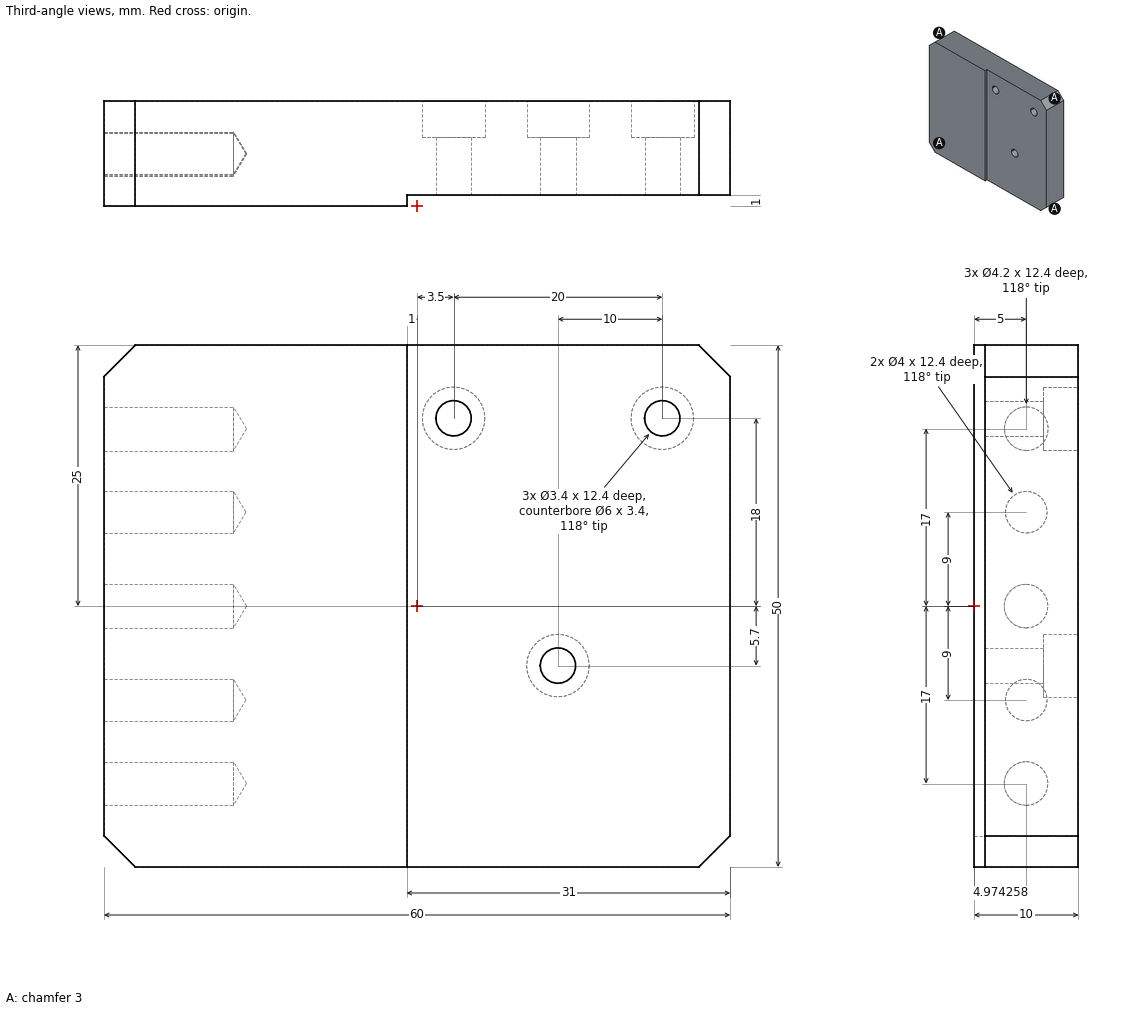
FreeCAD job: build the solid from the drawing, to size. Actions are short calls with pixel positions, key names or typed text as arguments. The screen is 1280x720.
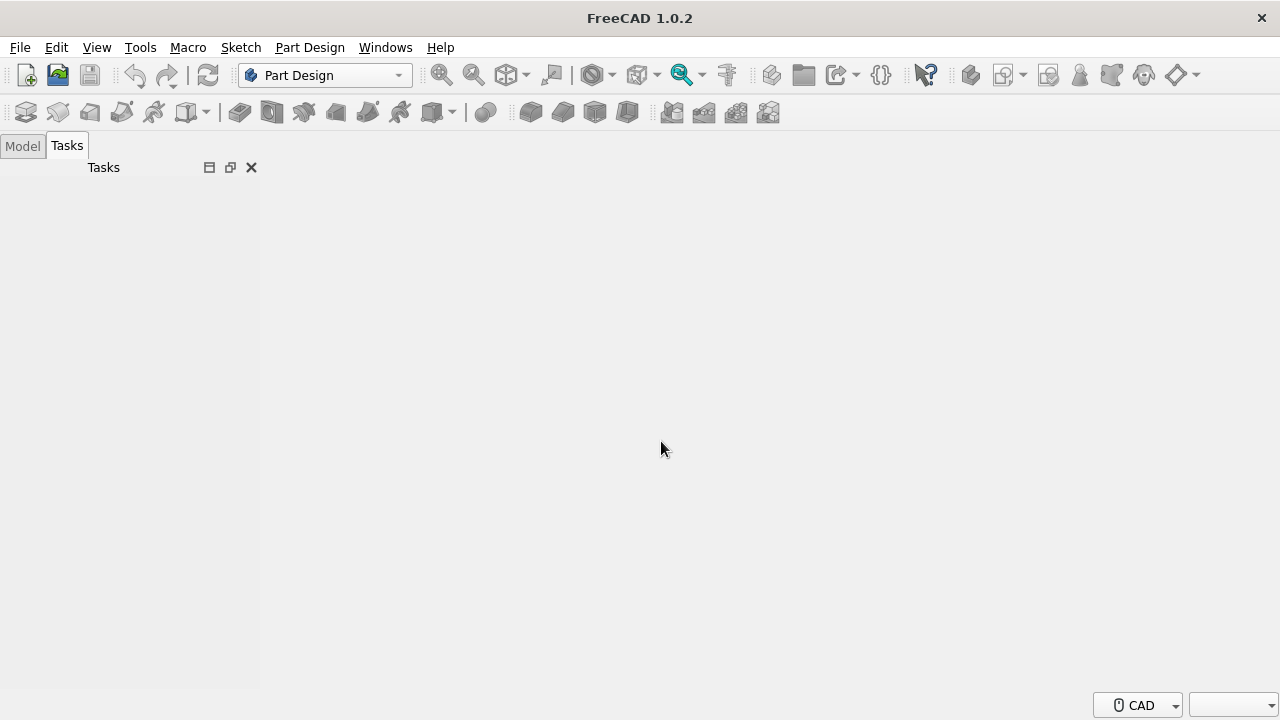
click(26, 76)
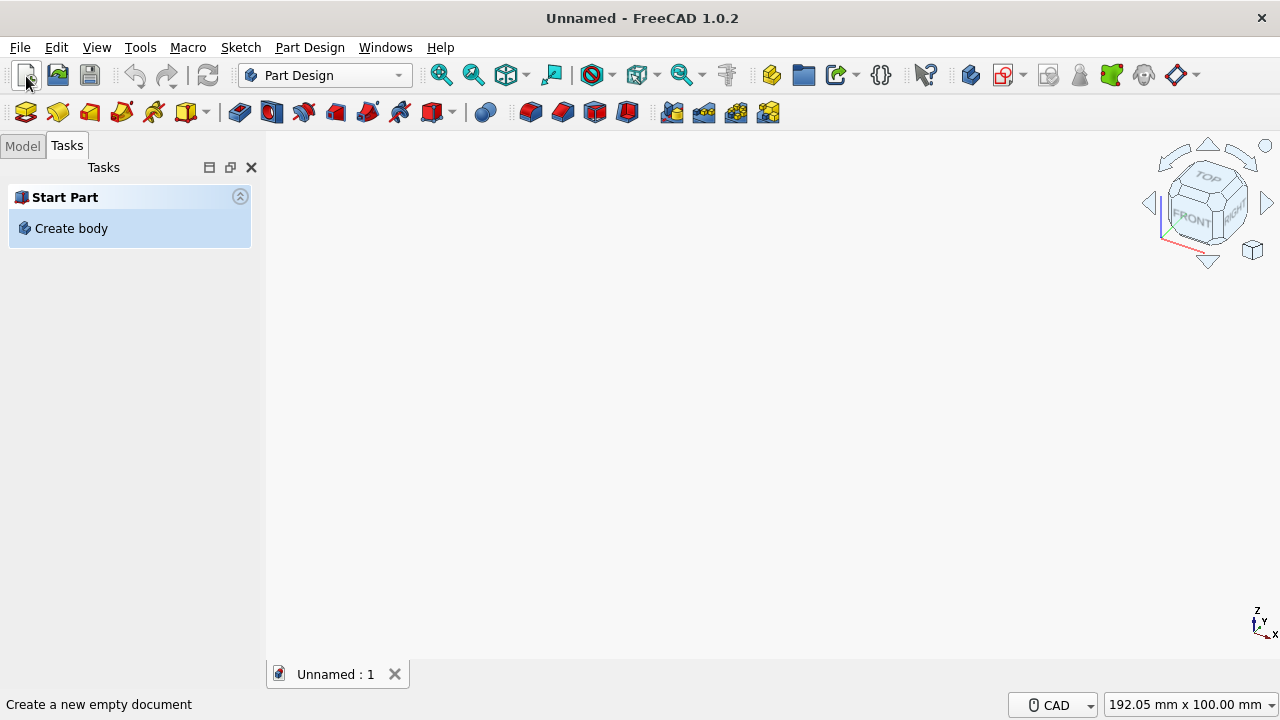
click(1004, 76)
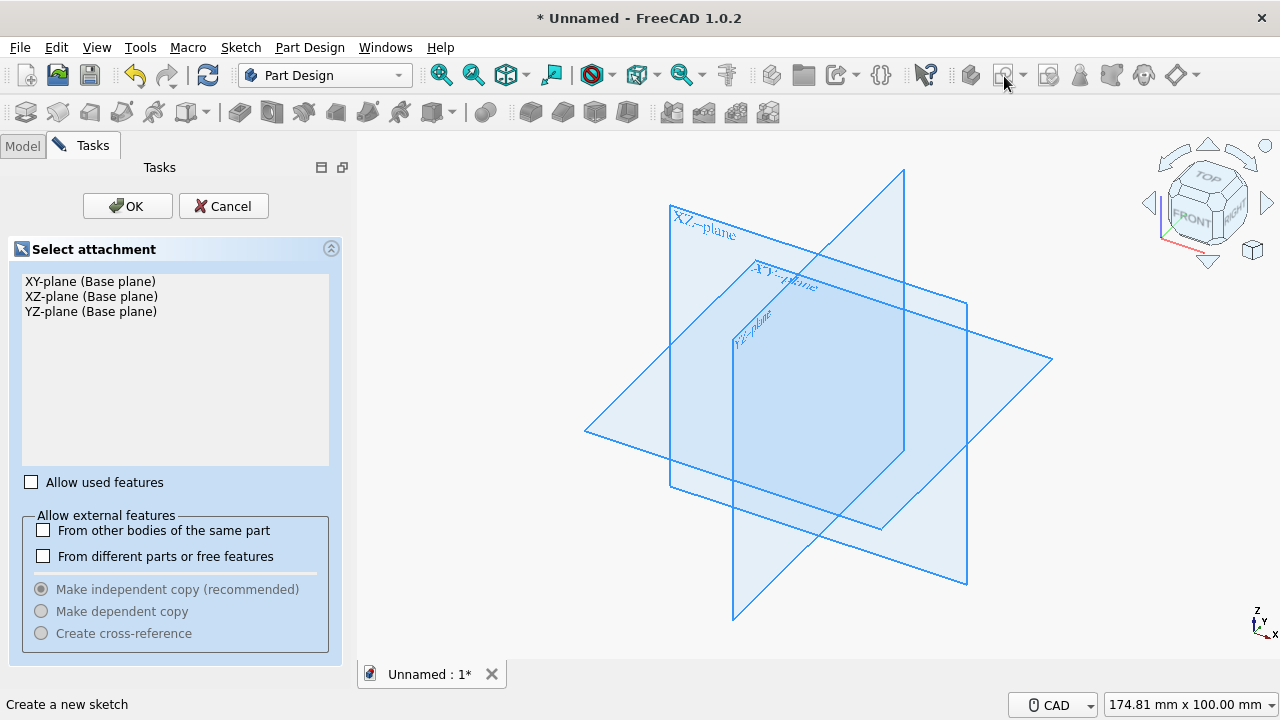
click(82, 296)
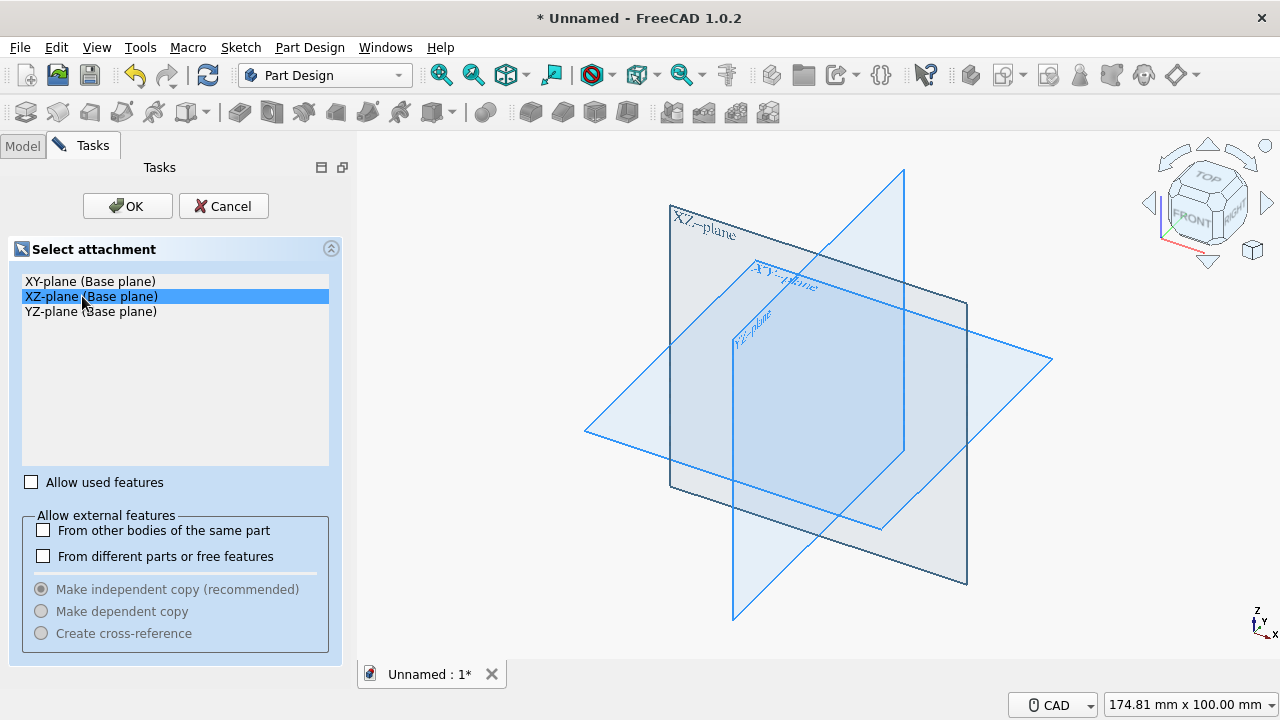
click(128, 206)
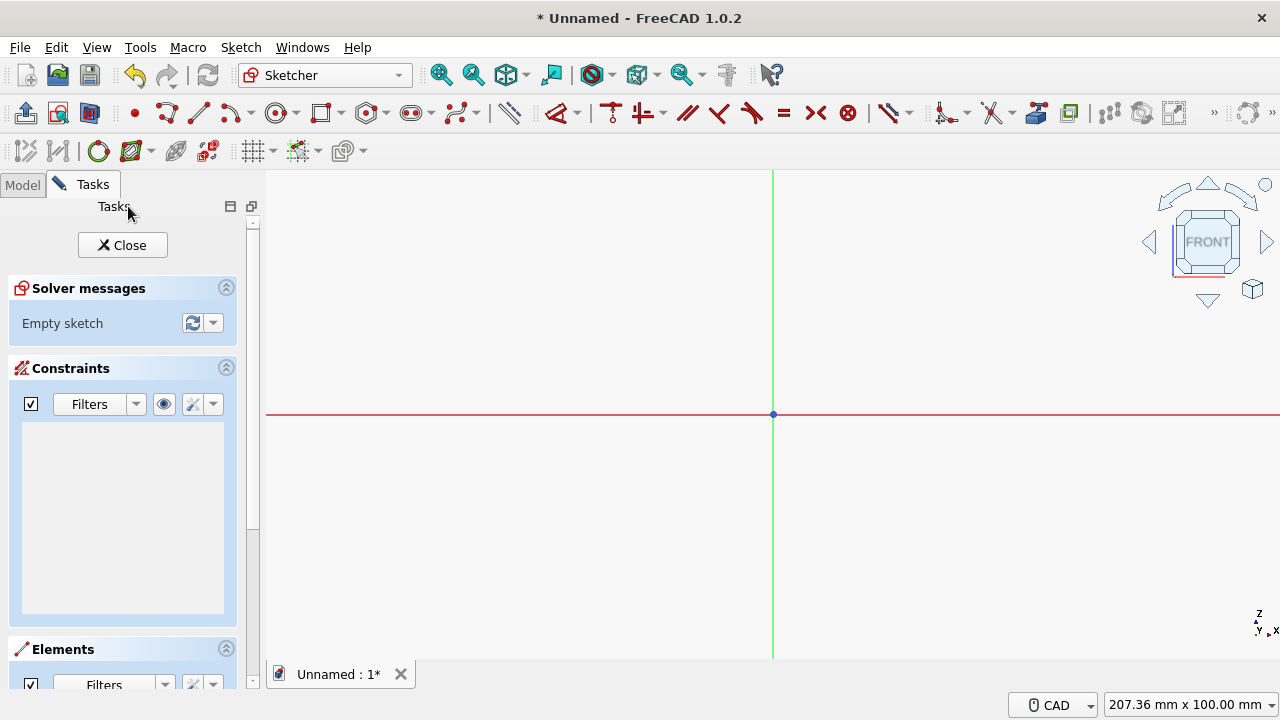
click(344, 114)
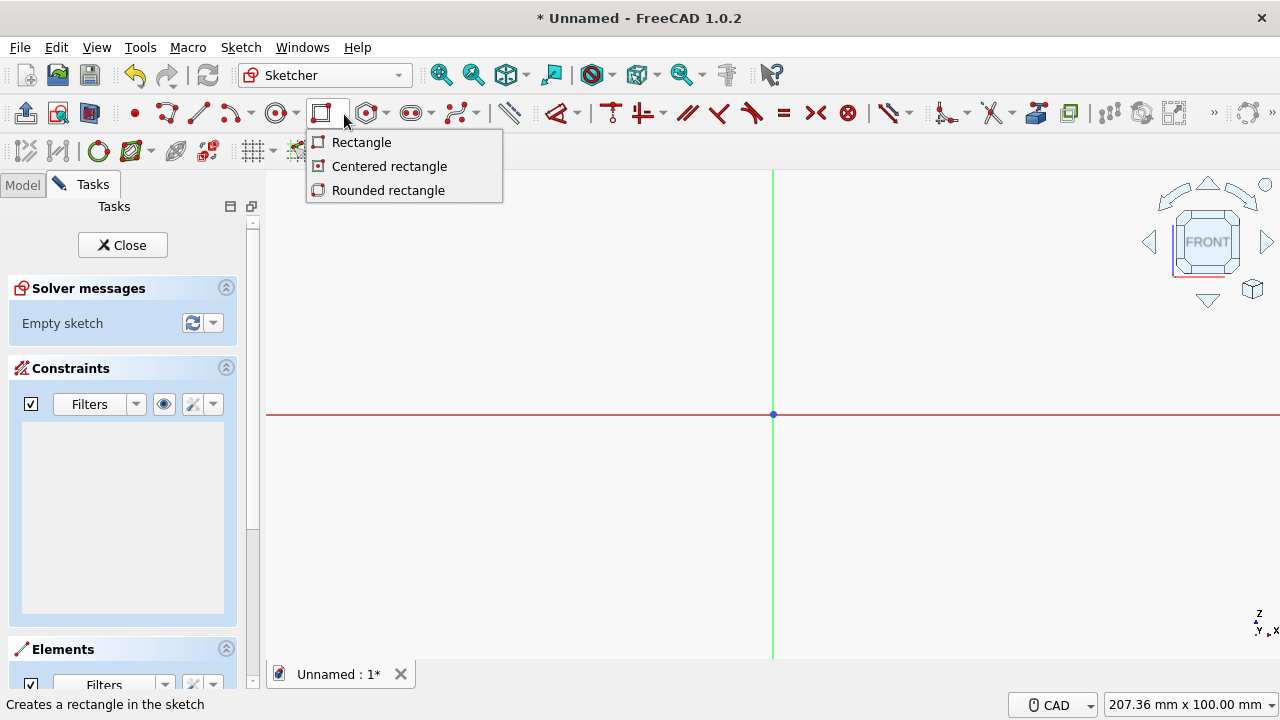
click(404, 166)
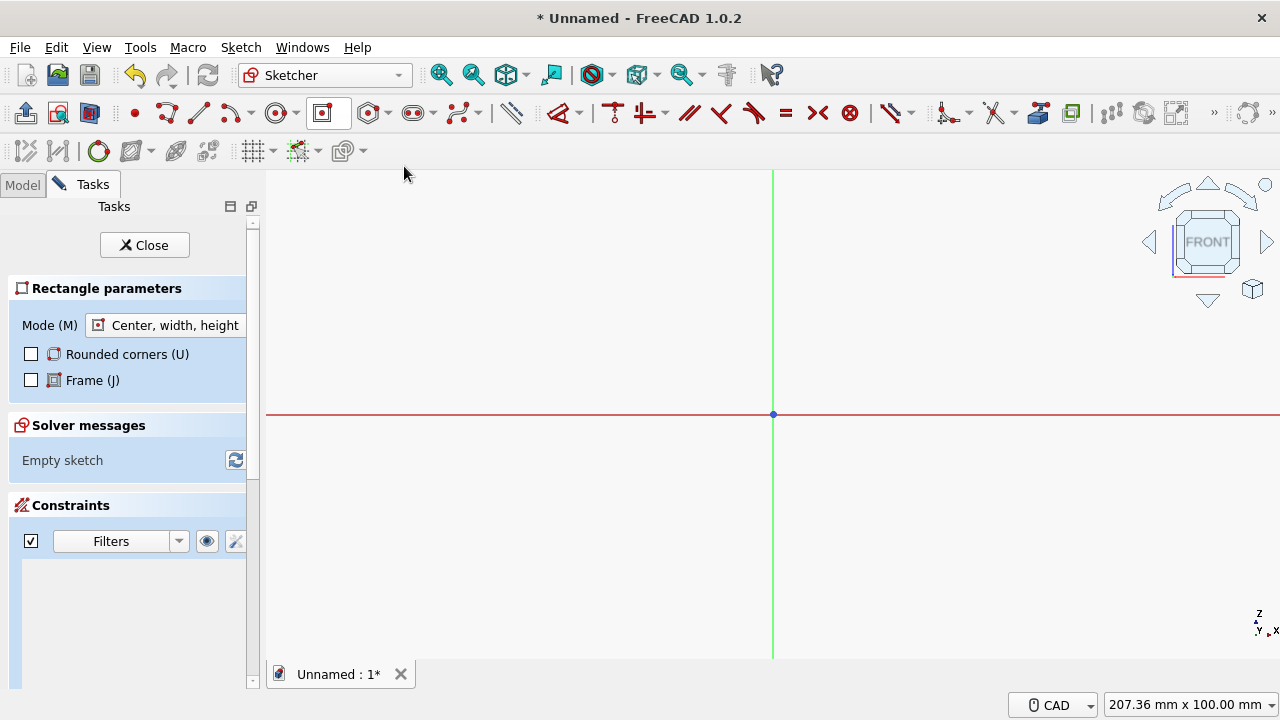
click(773, 414)
move(920, 292)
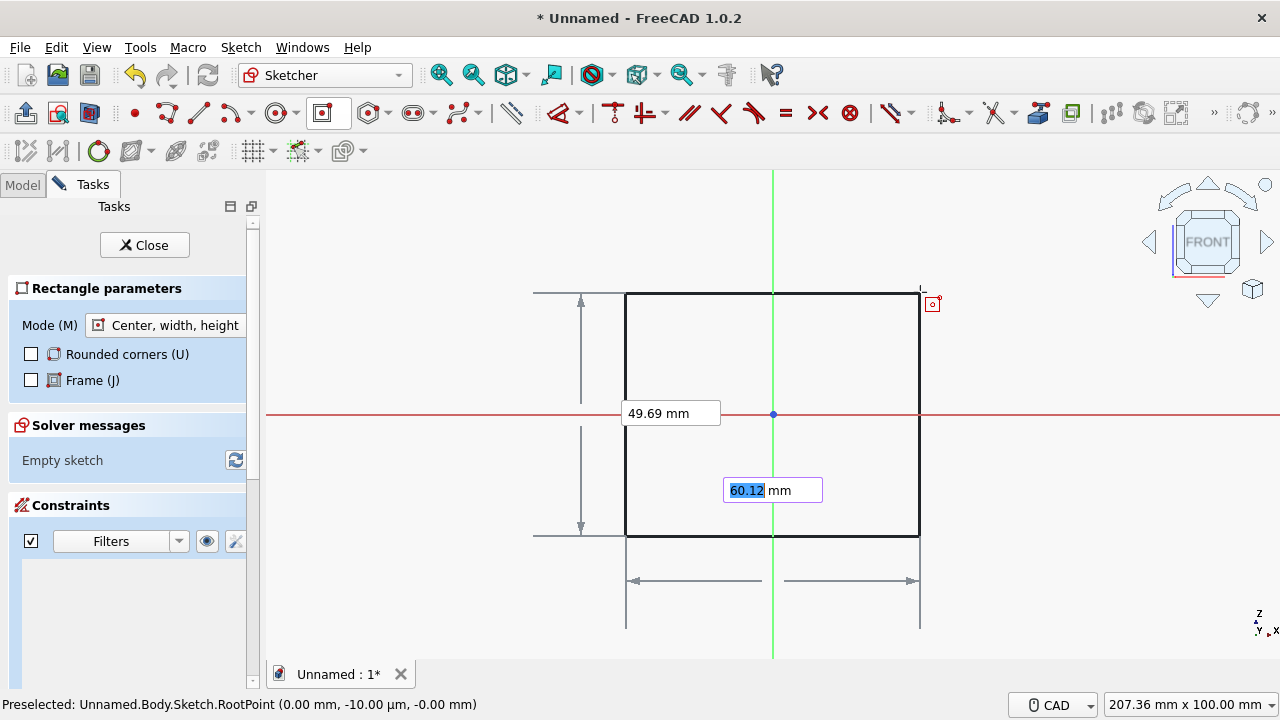
text(60)
key(Tab)
text(50)
key(Return)
key(Escape)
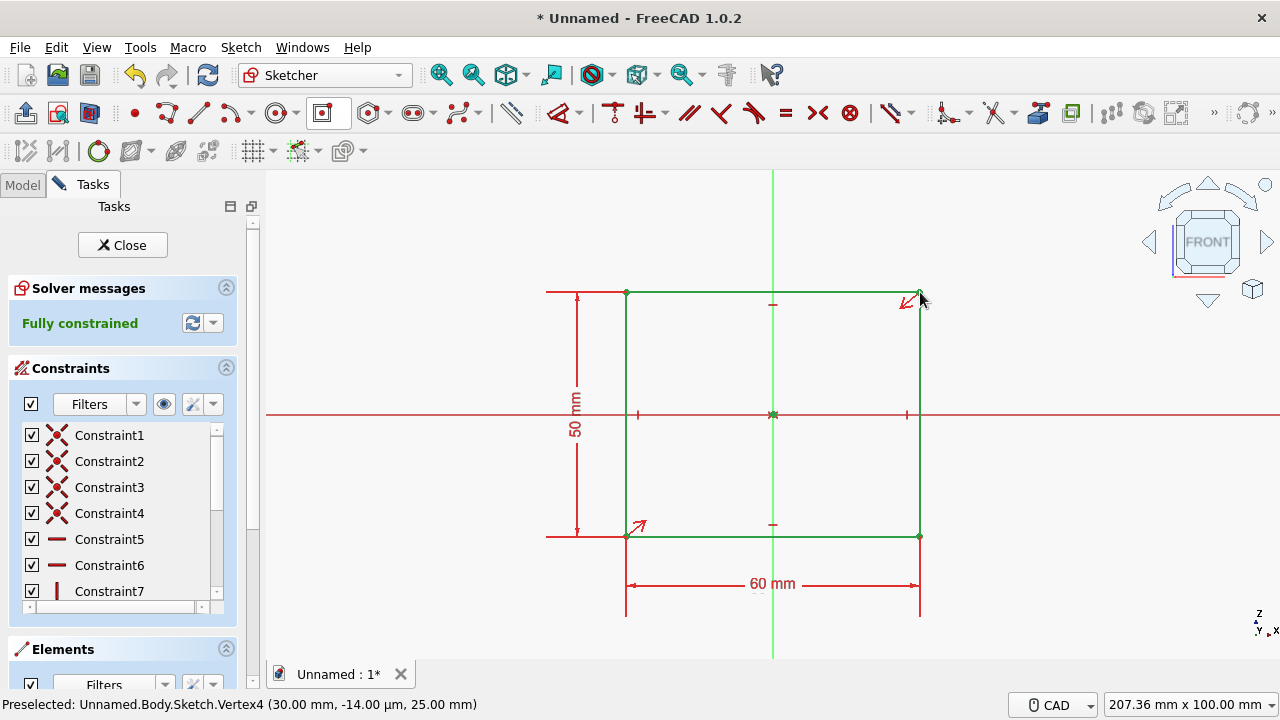
click(123, 245)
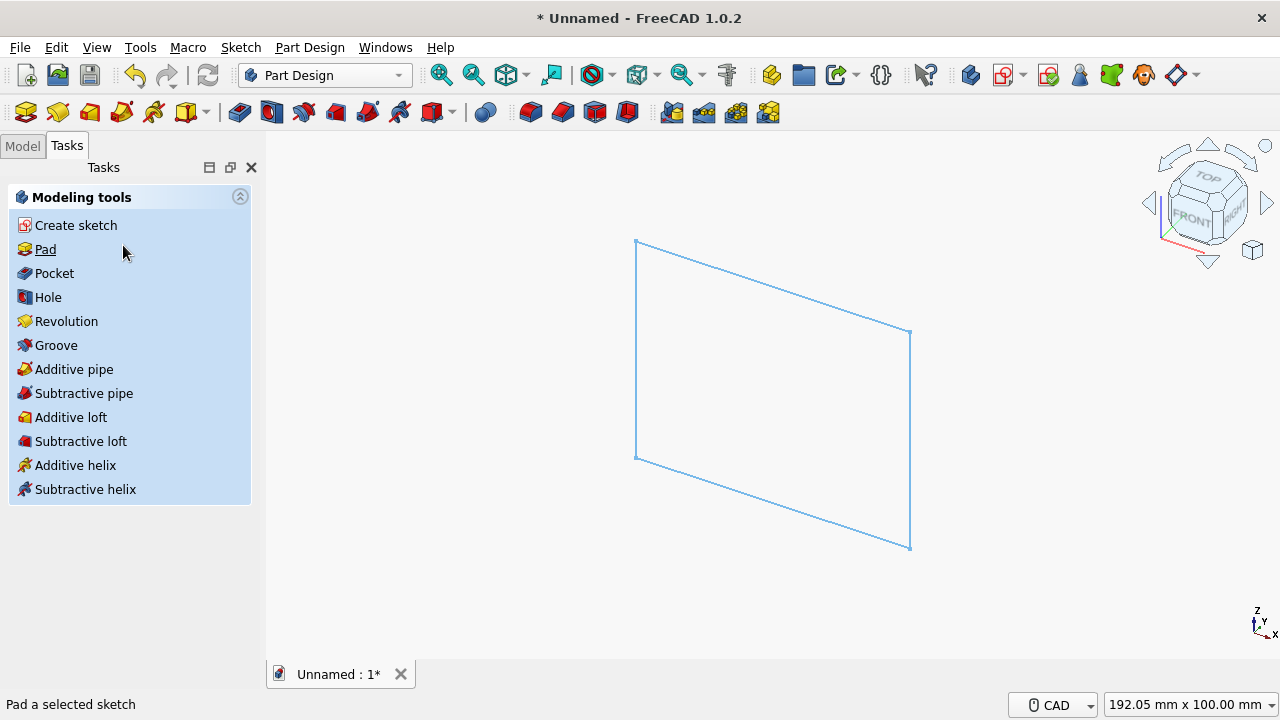
click(26, 112)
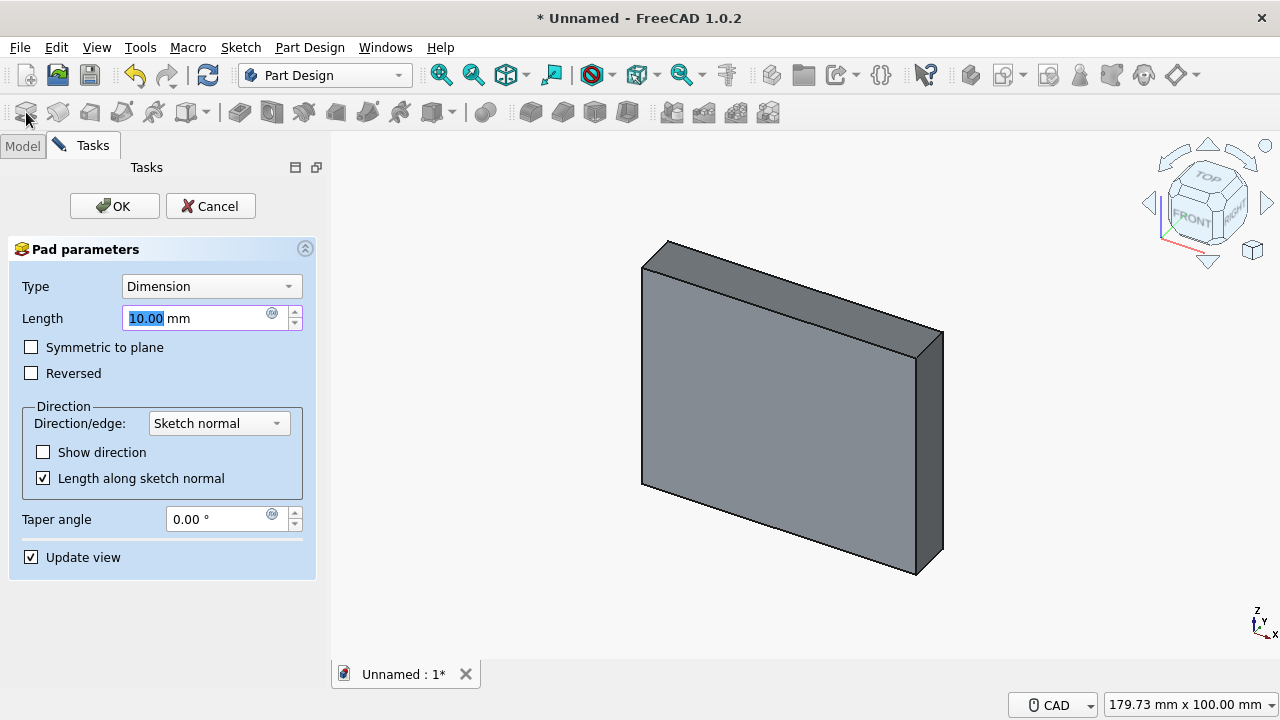
text(10)
key(Tab)